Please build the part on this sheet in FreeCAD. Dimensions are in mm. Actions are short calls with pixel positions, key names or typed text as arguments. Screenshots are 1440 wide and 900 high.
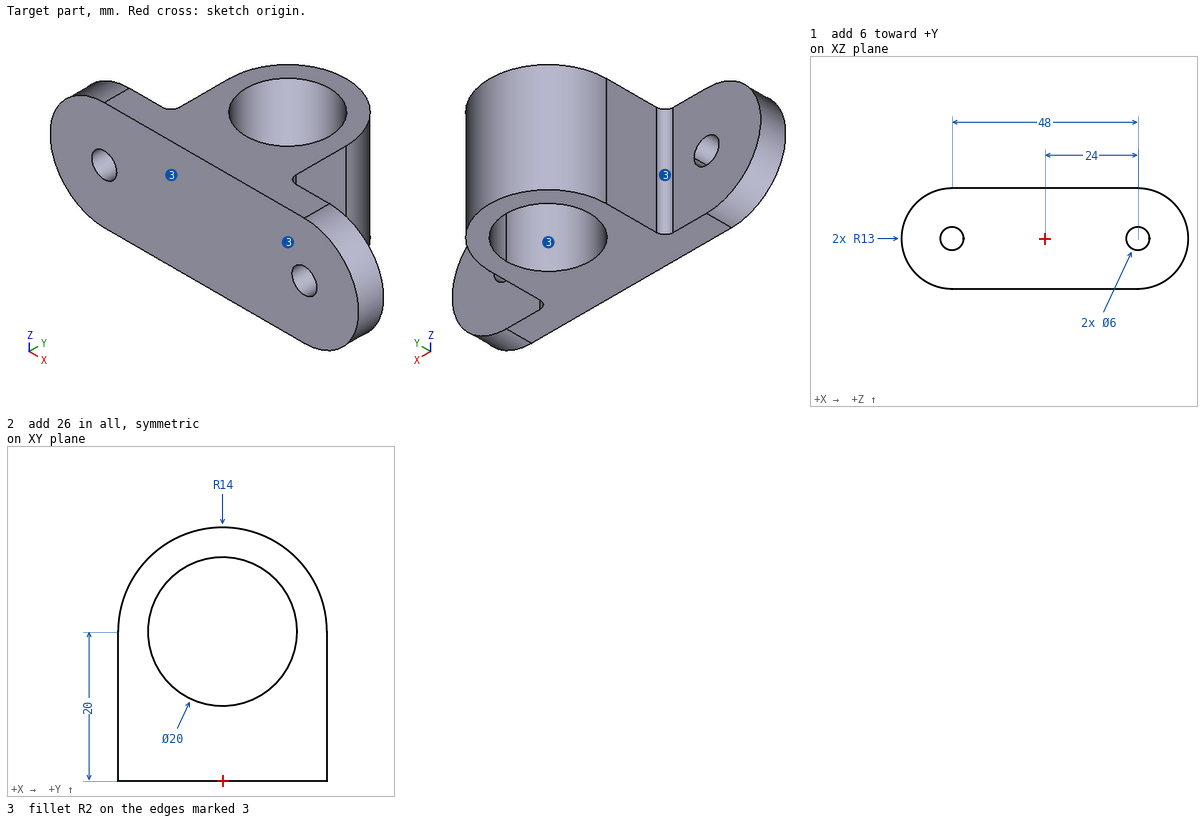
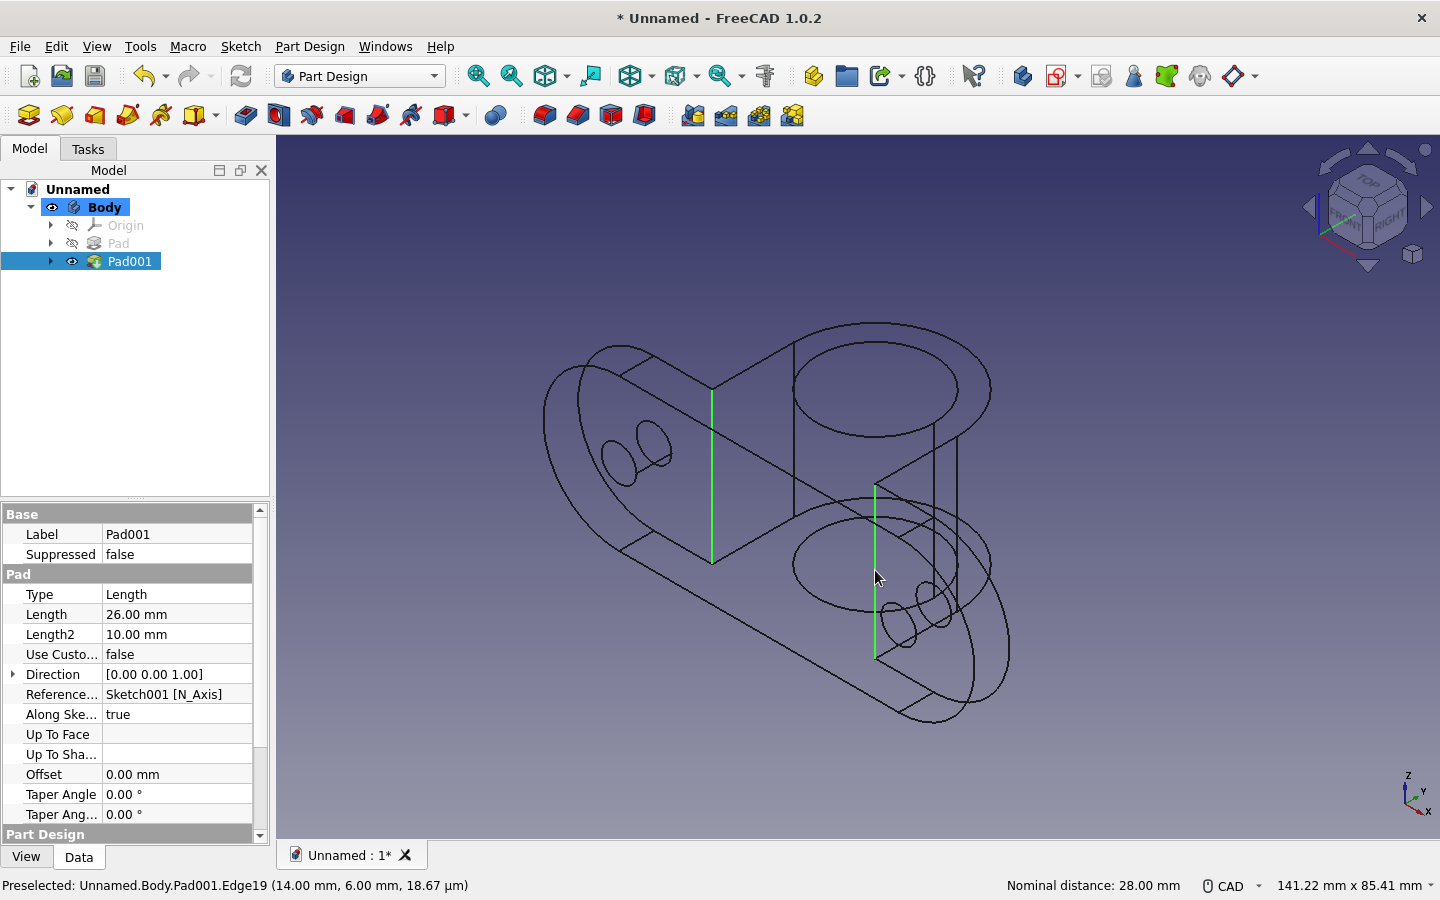
key(v)
key(1)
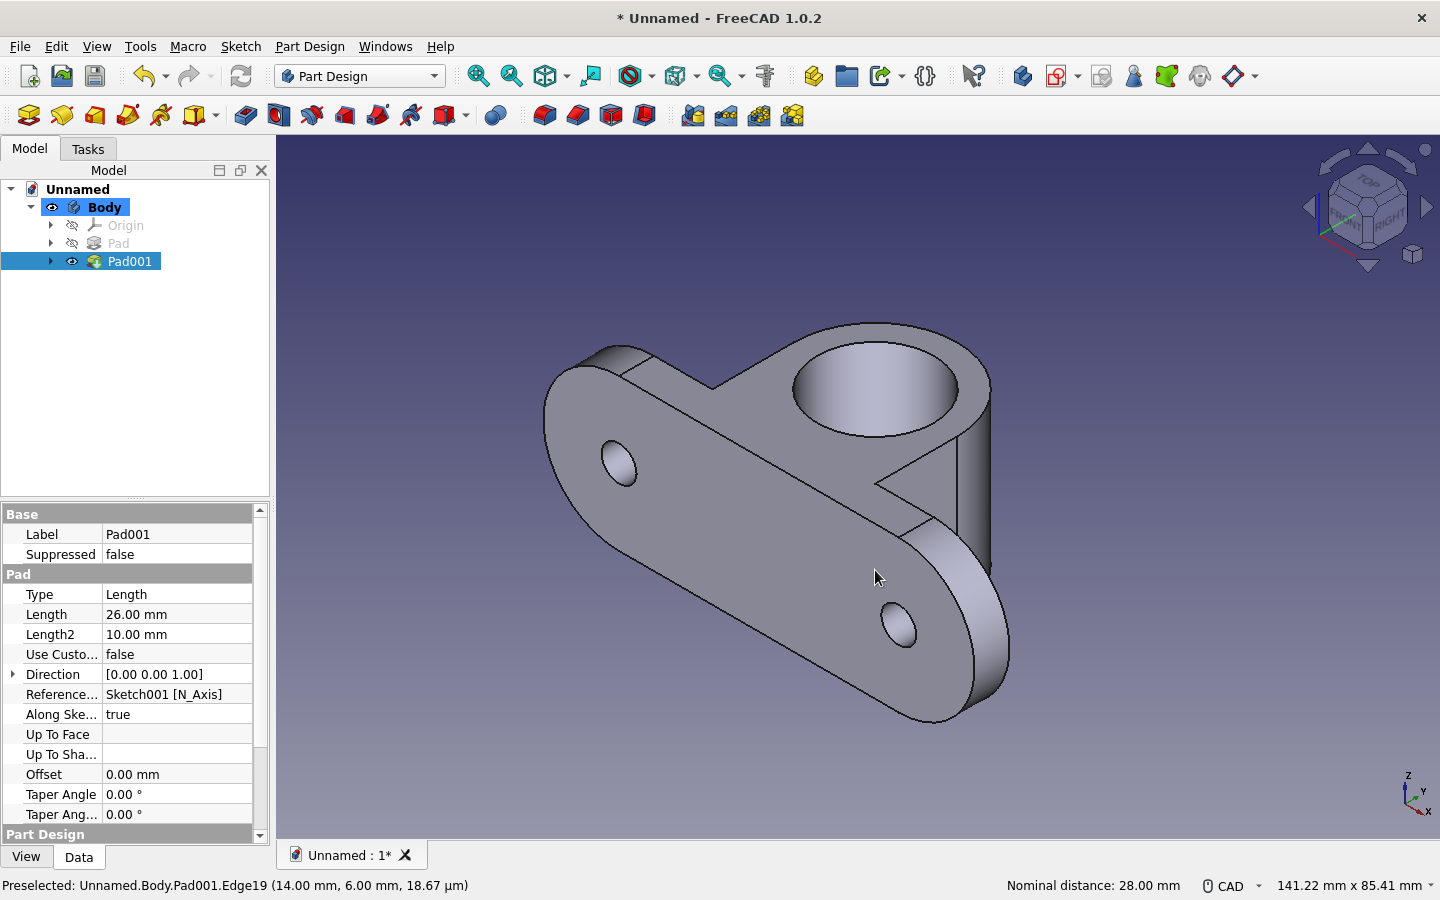
click(545, 116)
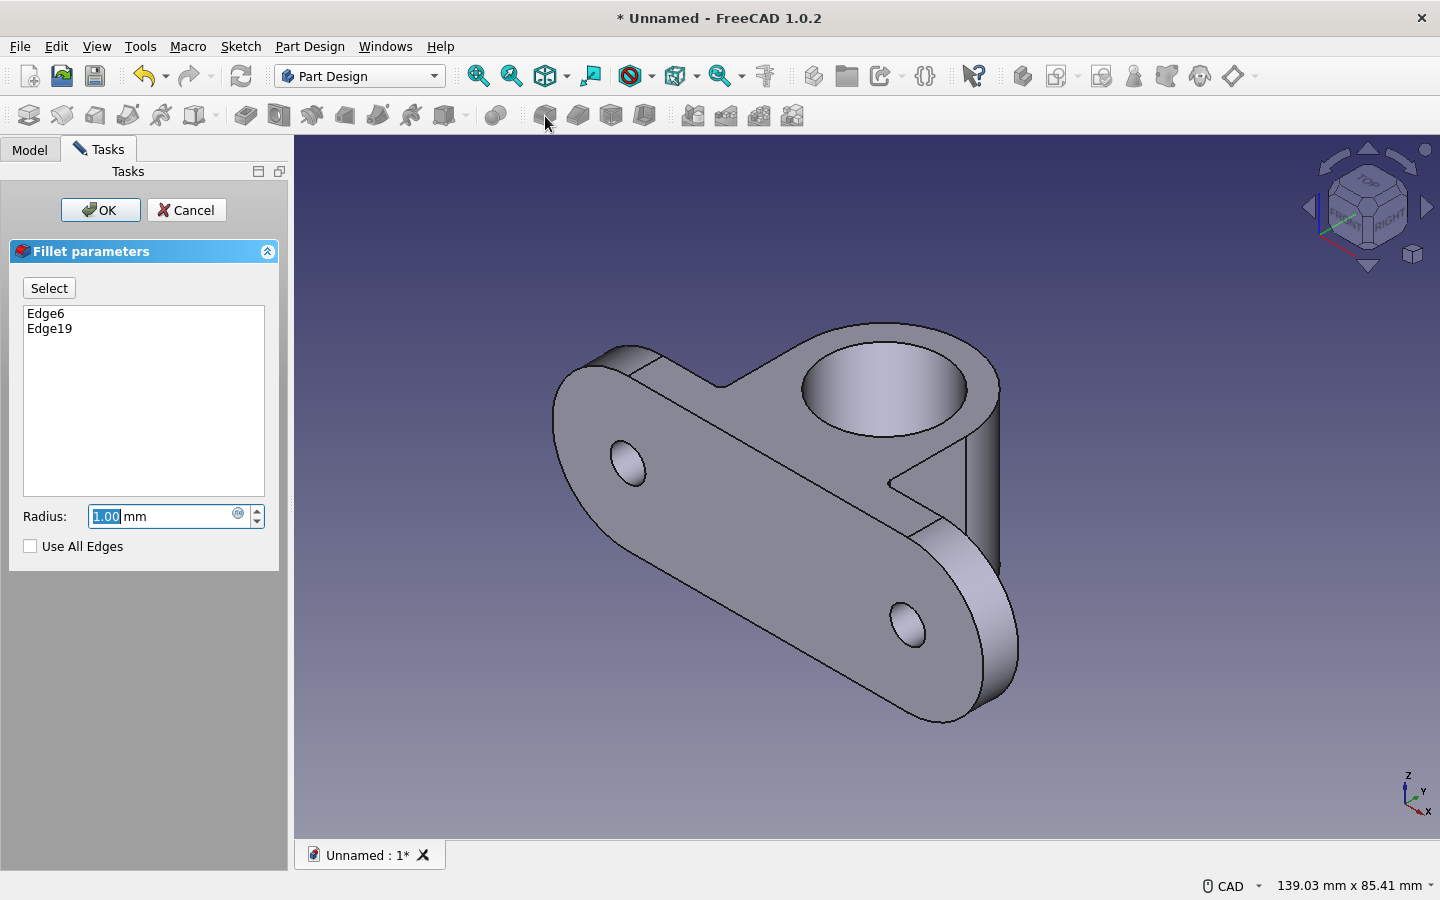
text(2)
key(Tab)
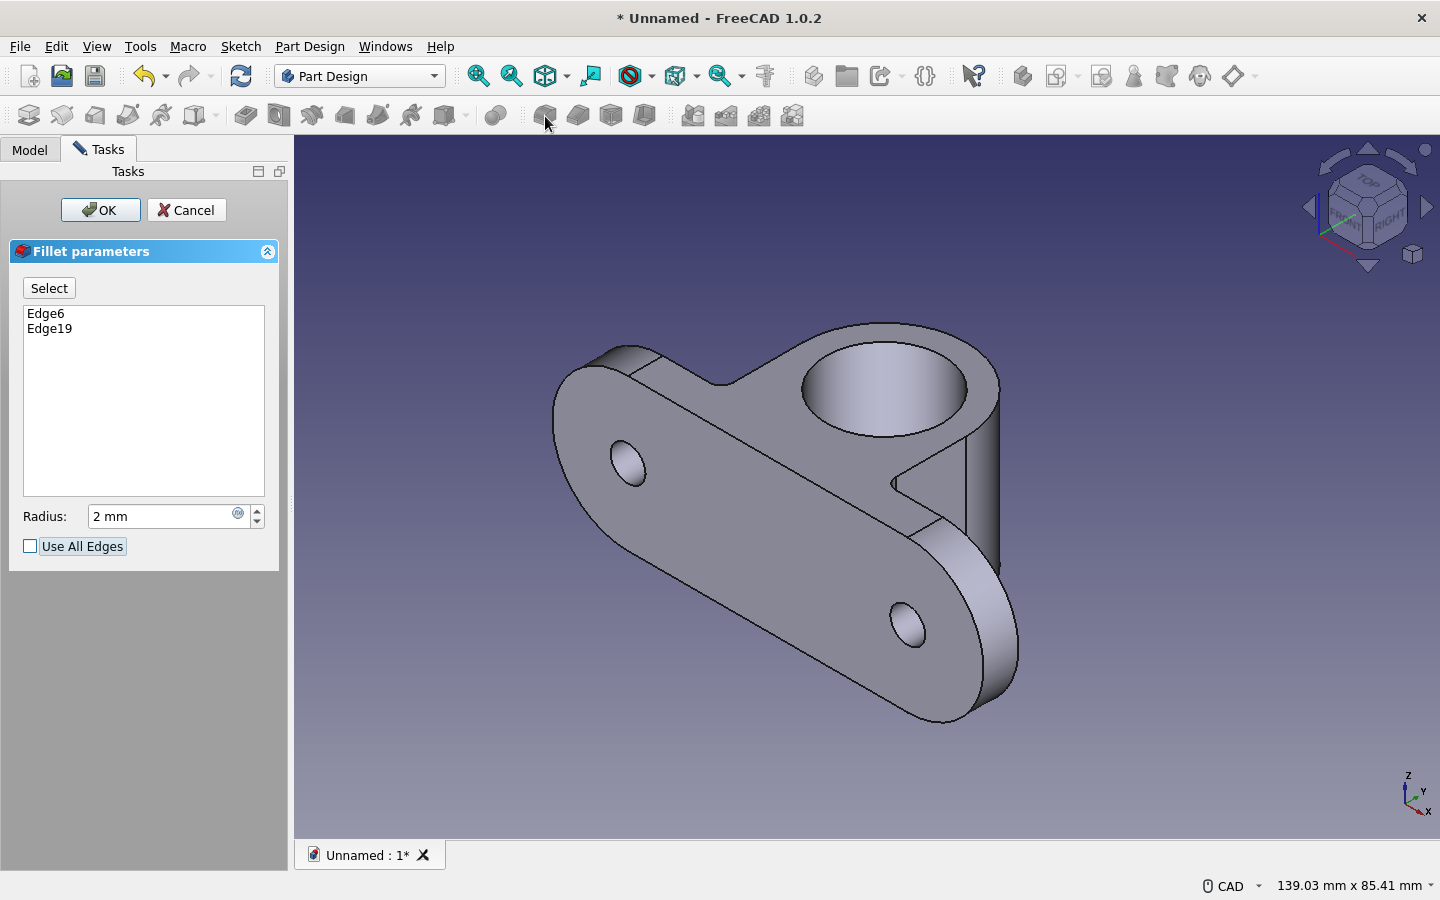
click(101, 210)